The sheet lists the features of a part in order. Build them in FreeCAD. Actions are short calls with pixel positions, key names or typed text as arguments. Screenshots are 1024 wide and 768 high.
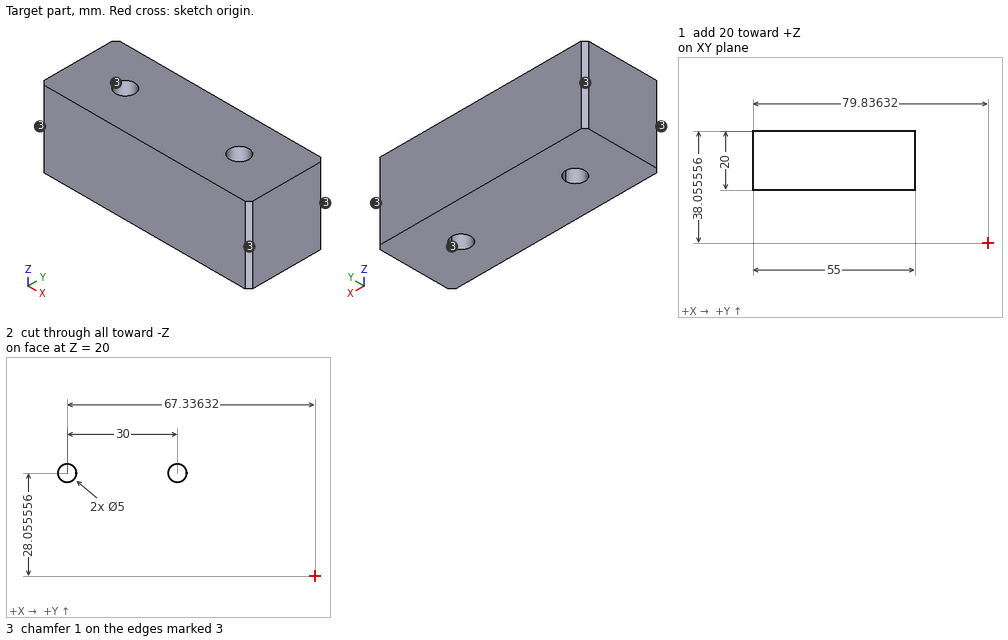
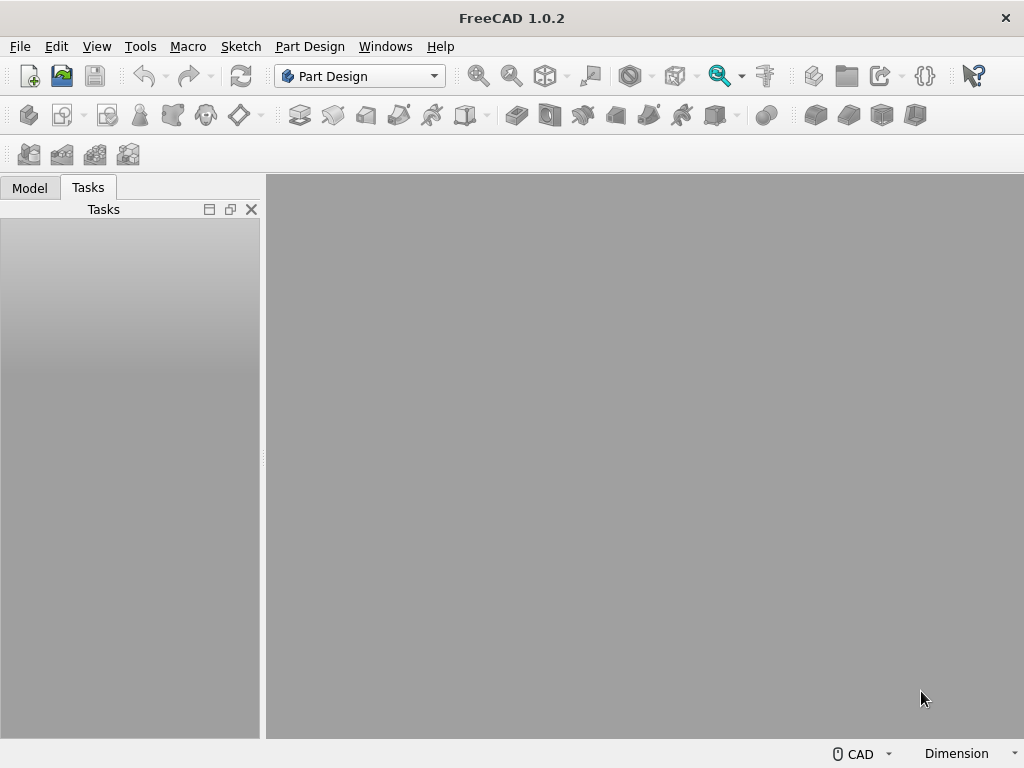
click(29, 76)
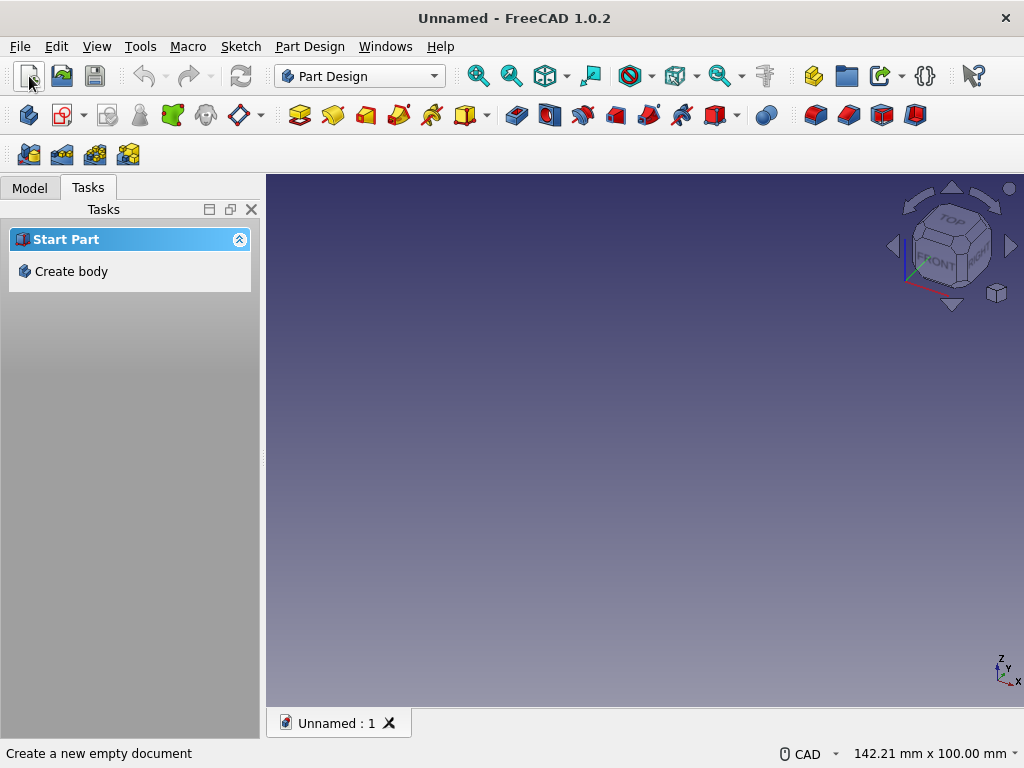
click(62, 116)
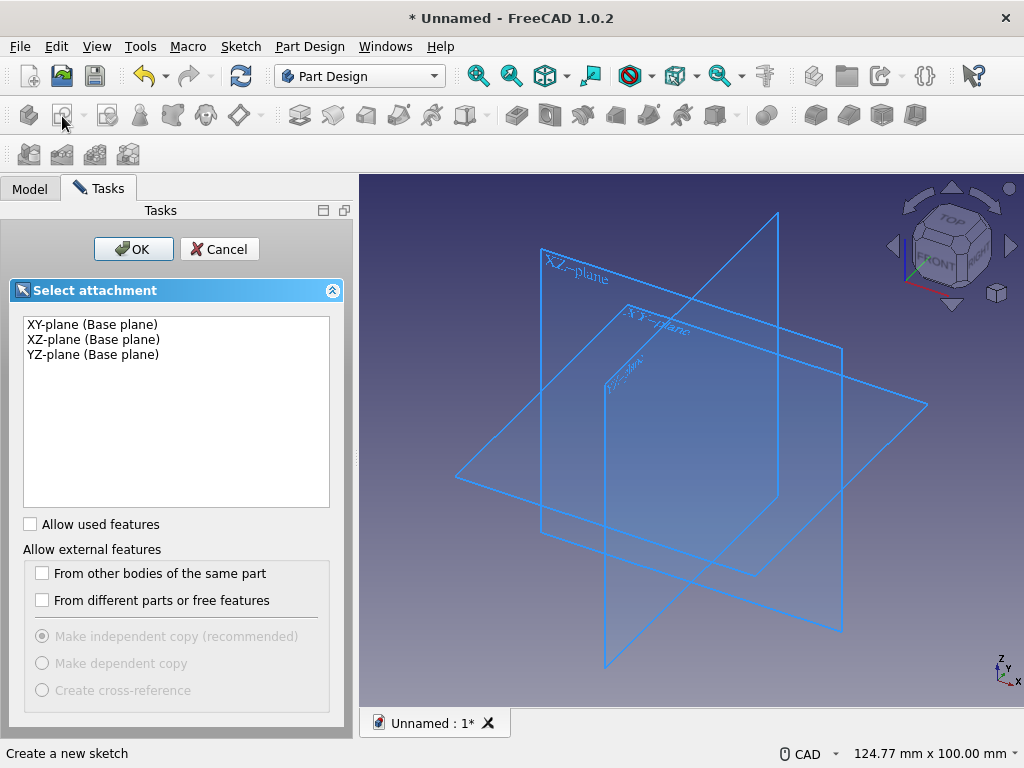
click(84, 324)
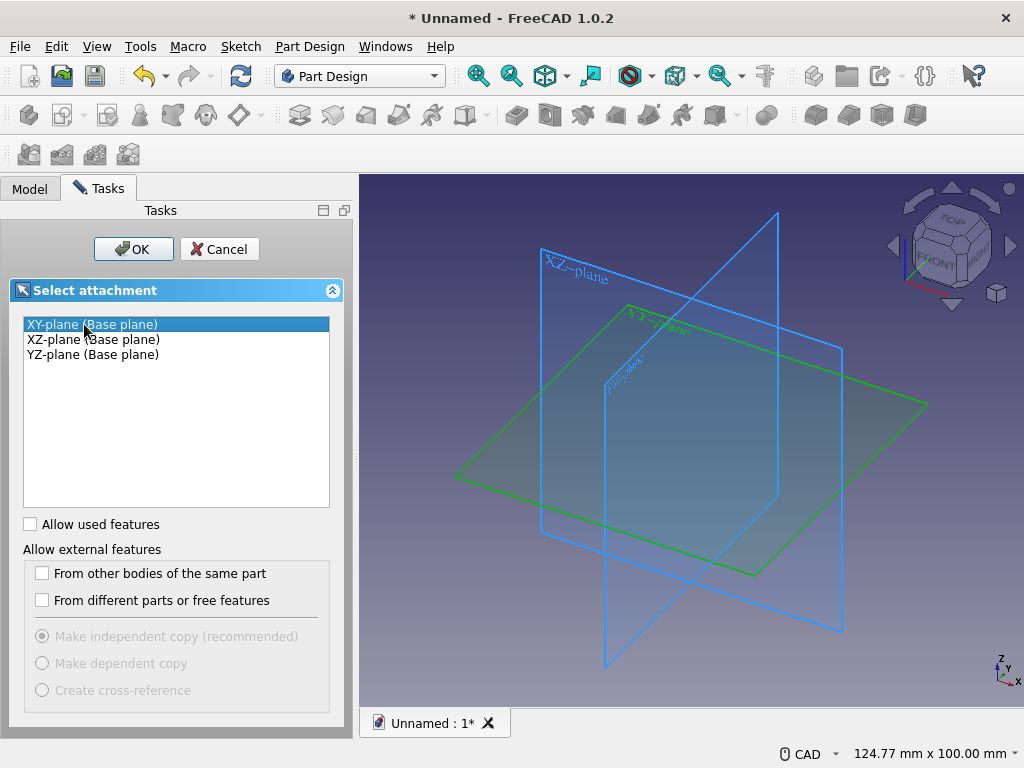
click(134, 249)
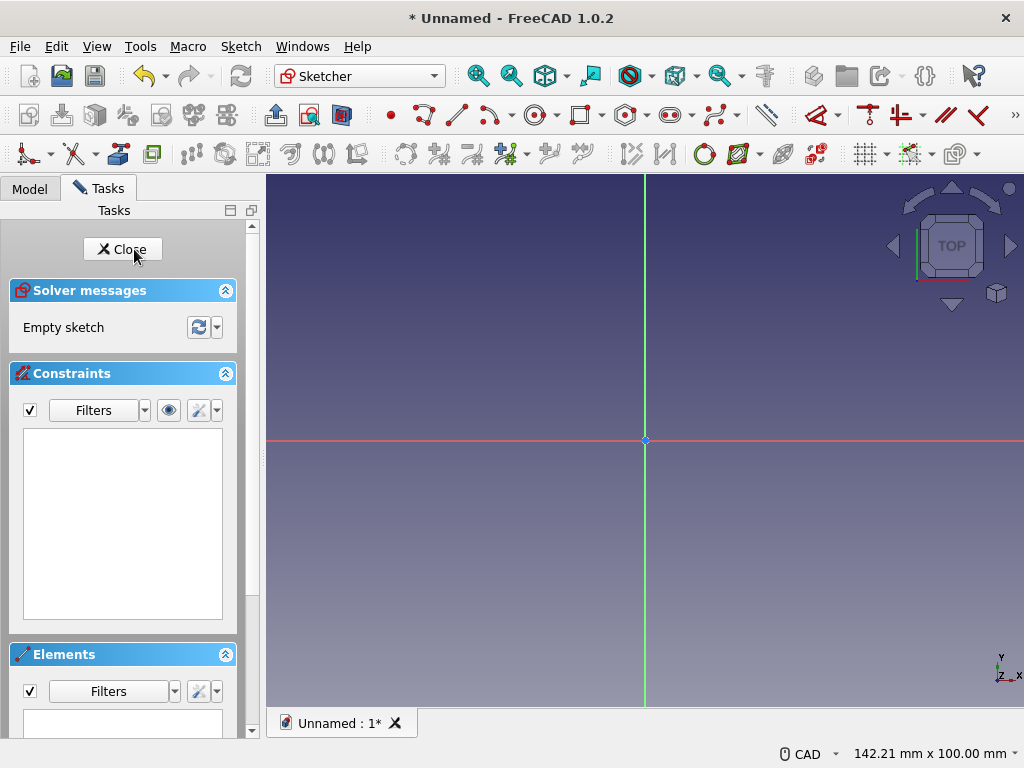
scroll(859, 679, down, 1)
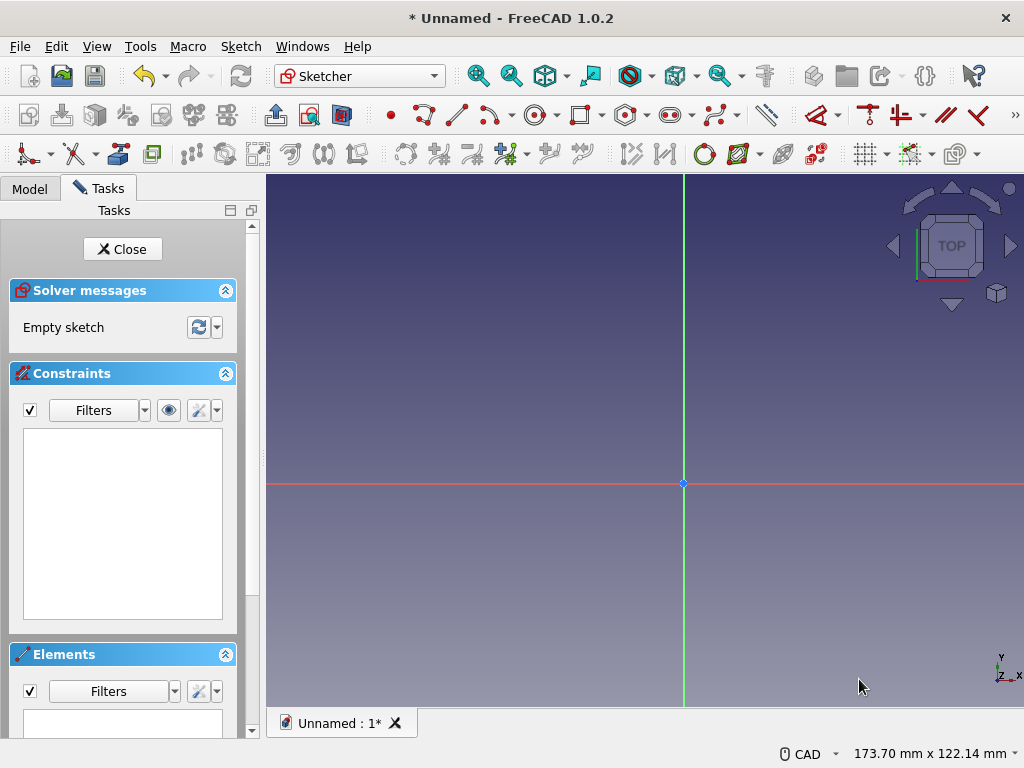
click(580, 116)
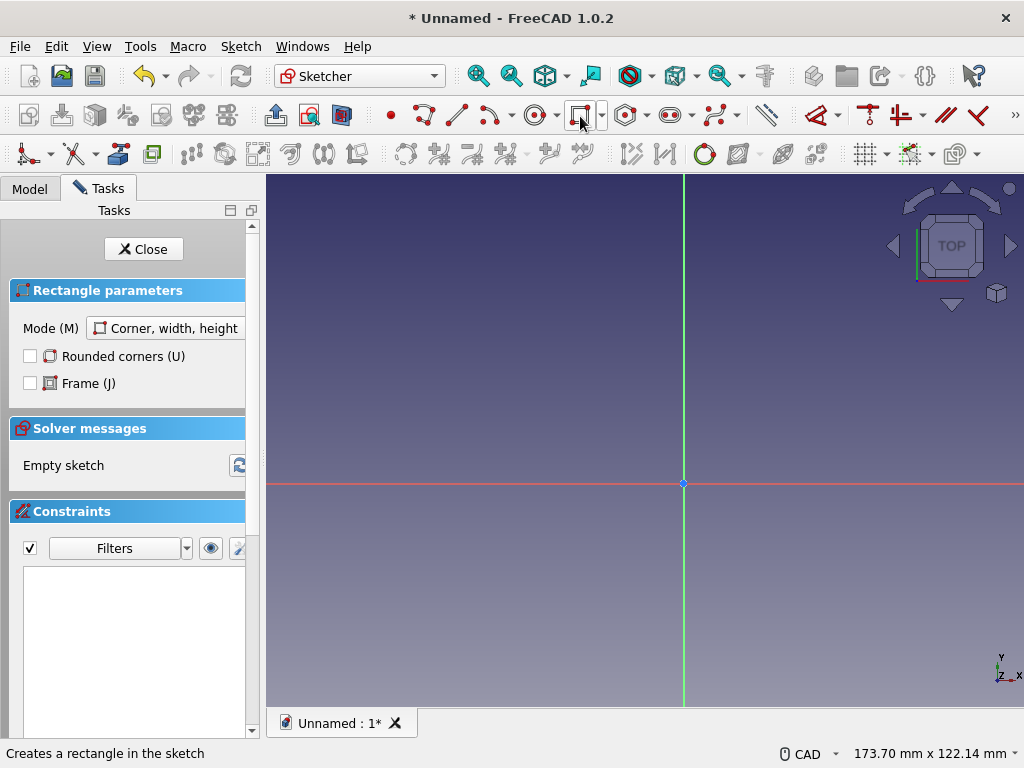
click(336, 318)
click(576, 405)
key(Escape)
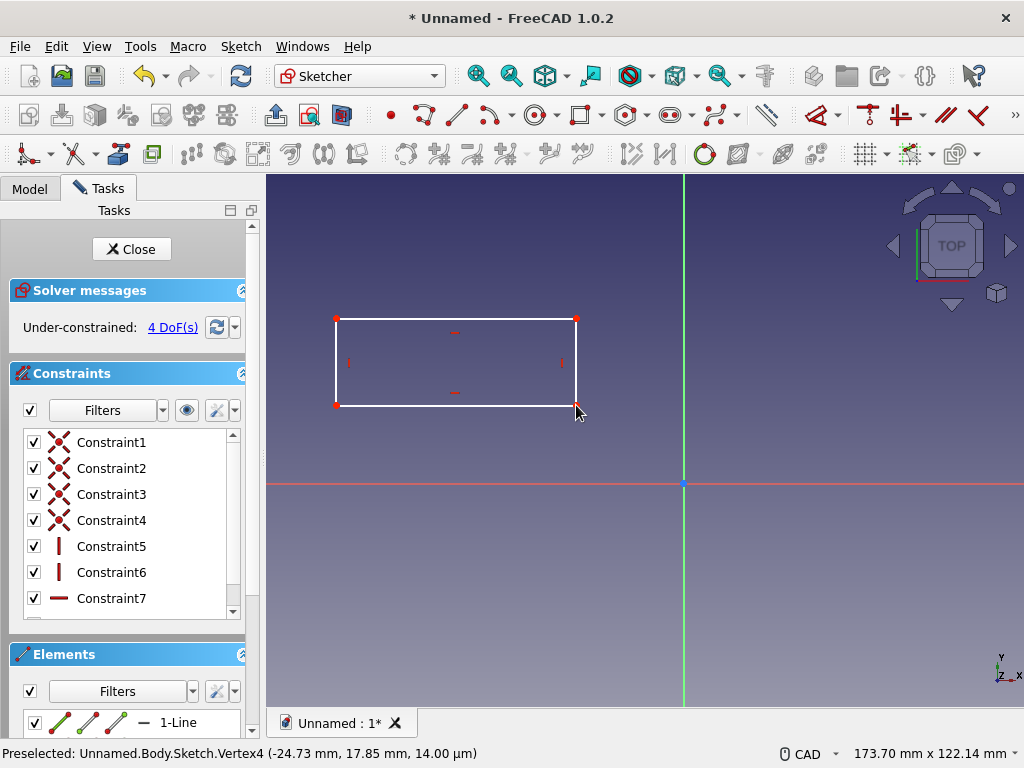
click(336, 345)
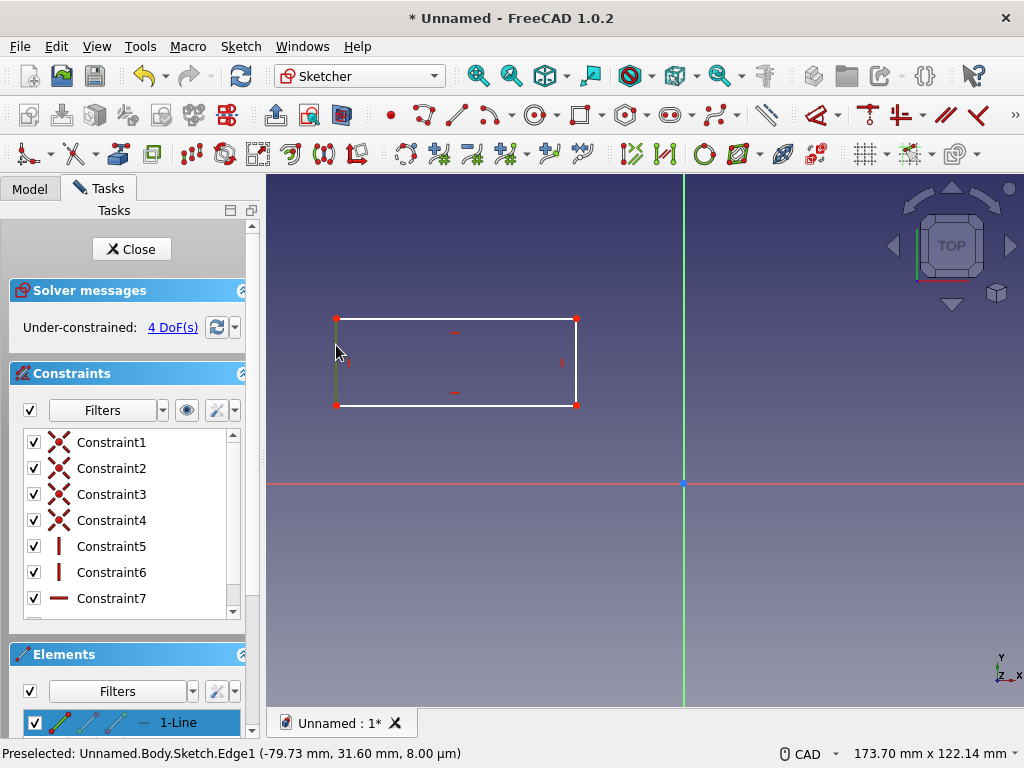
key(i)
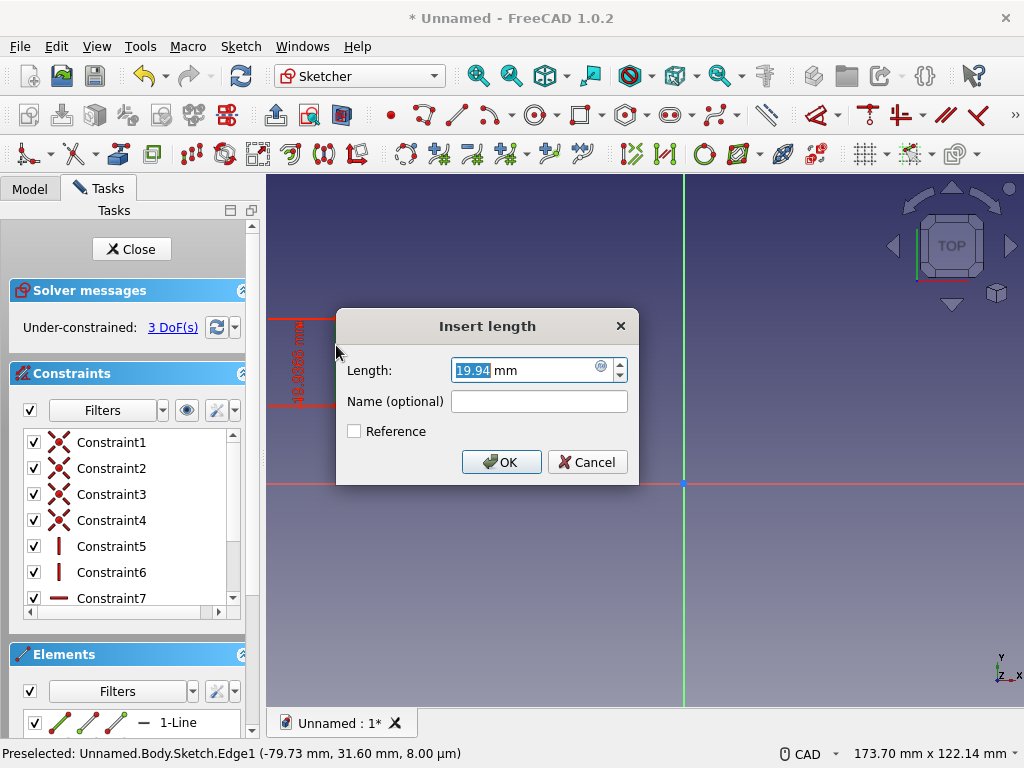
text(20)
key(Return)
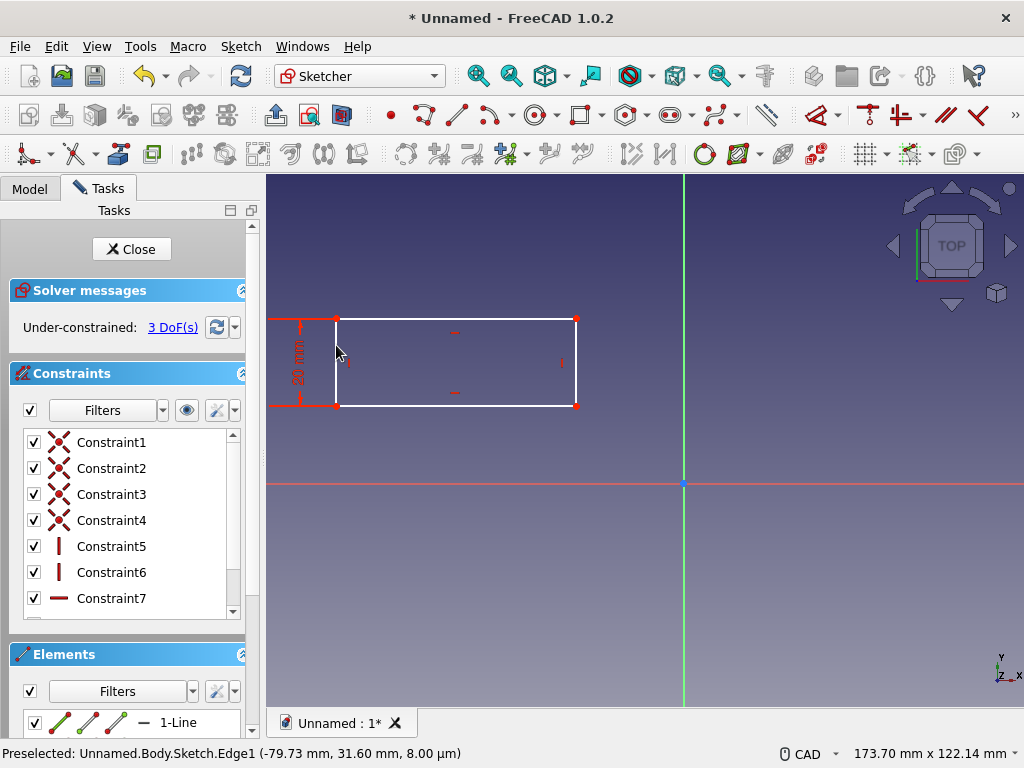
click(408, 406)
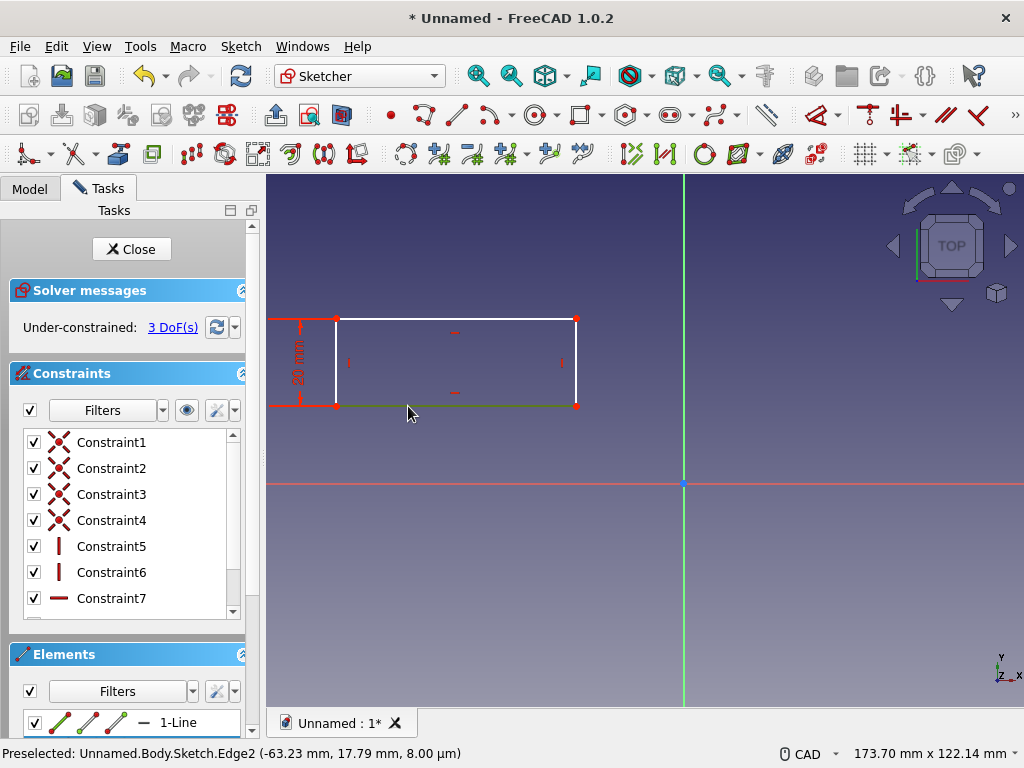
key(l)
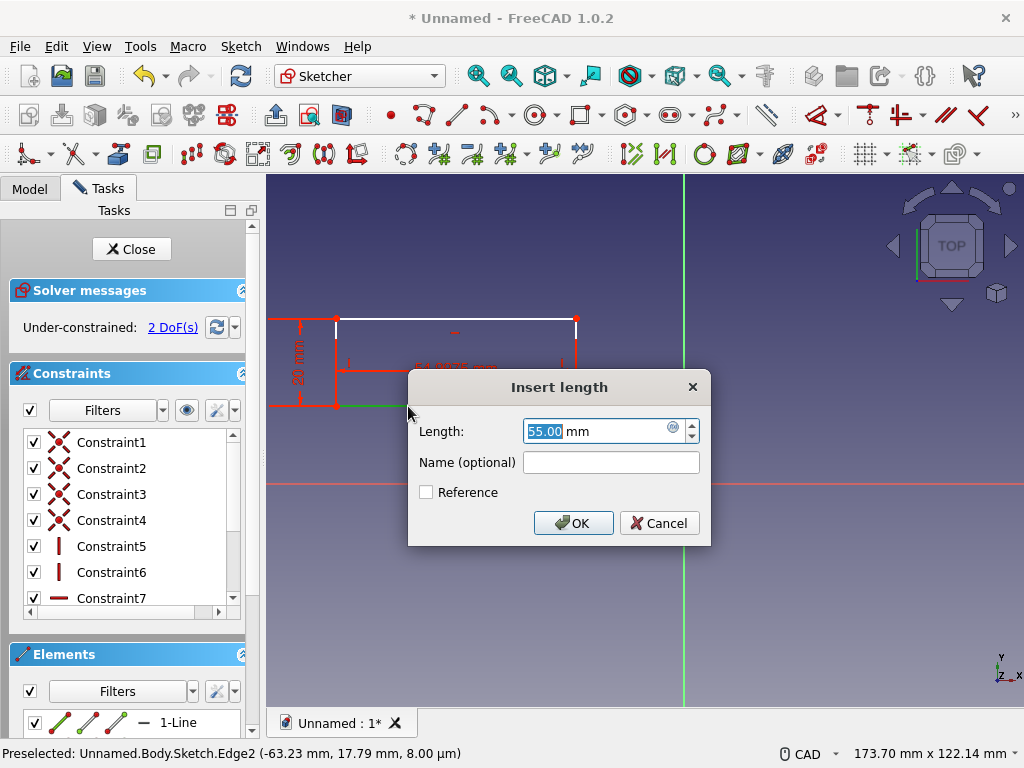
text(55)
key(Return)